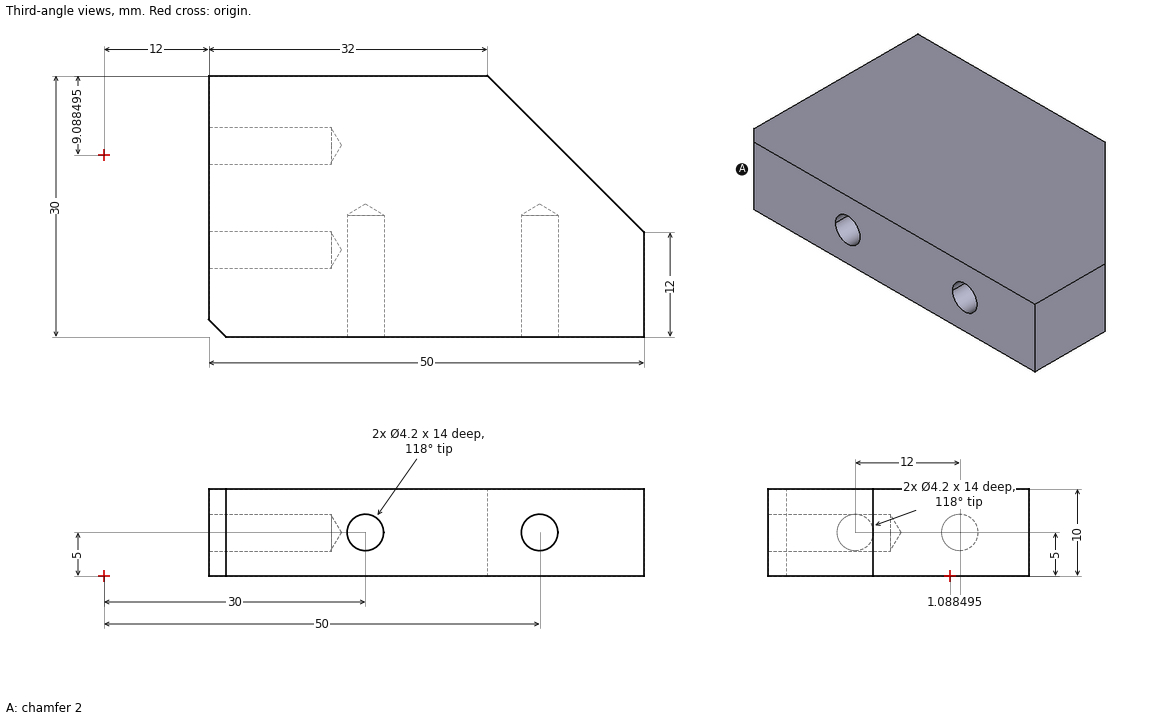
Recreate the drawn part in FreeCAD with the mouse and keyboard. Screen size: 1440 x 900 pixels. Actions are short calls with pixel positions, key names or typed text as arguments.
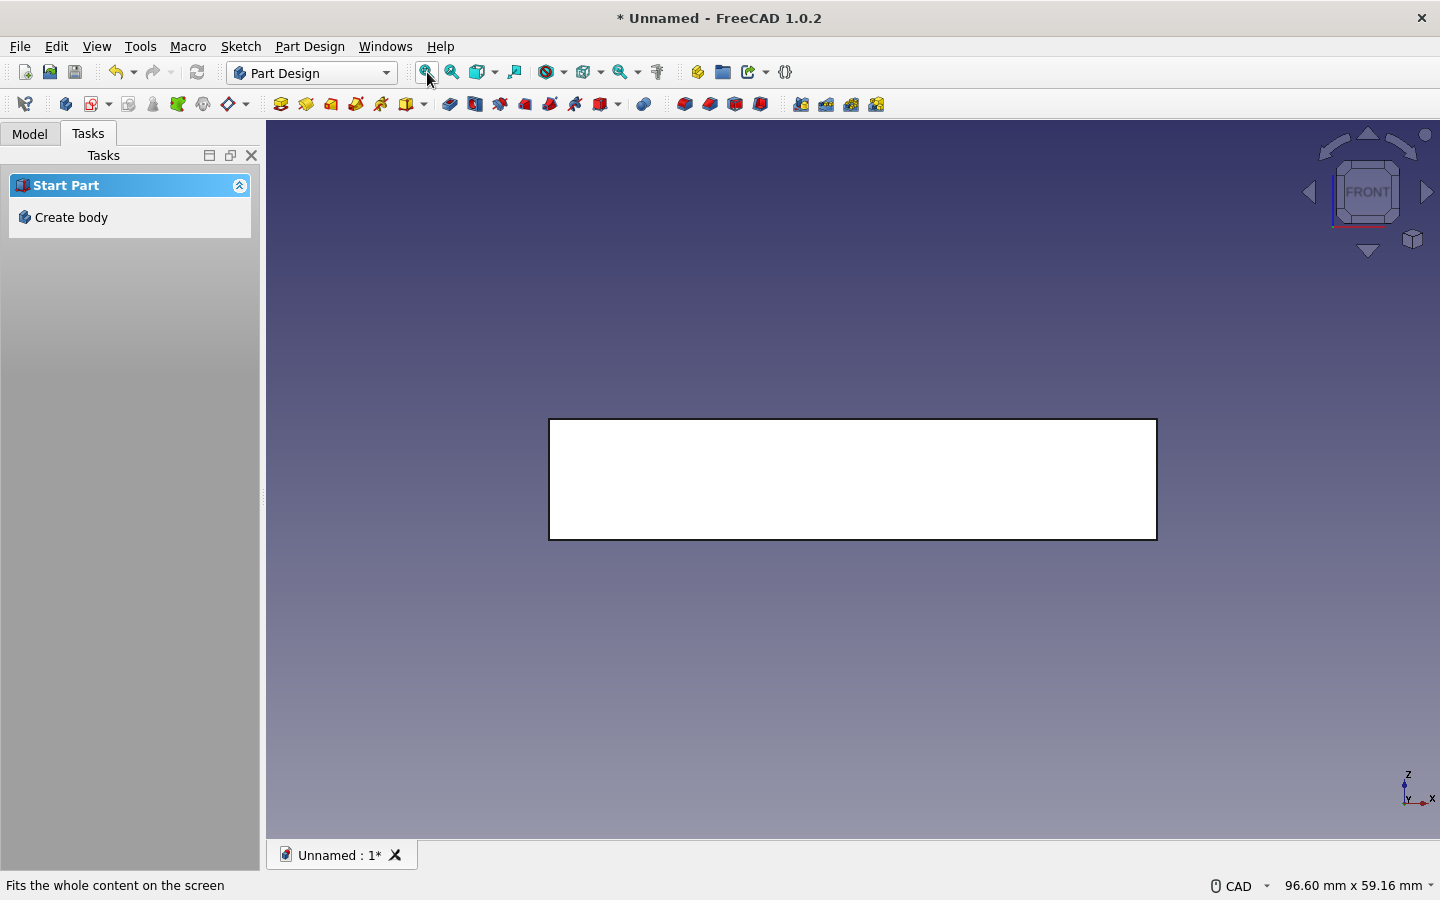
click(549, 479)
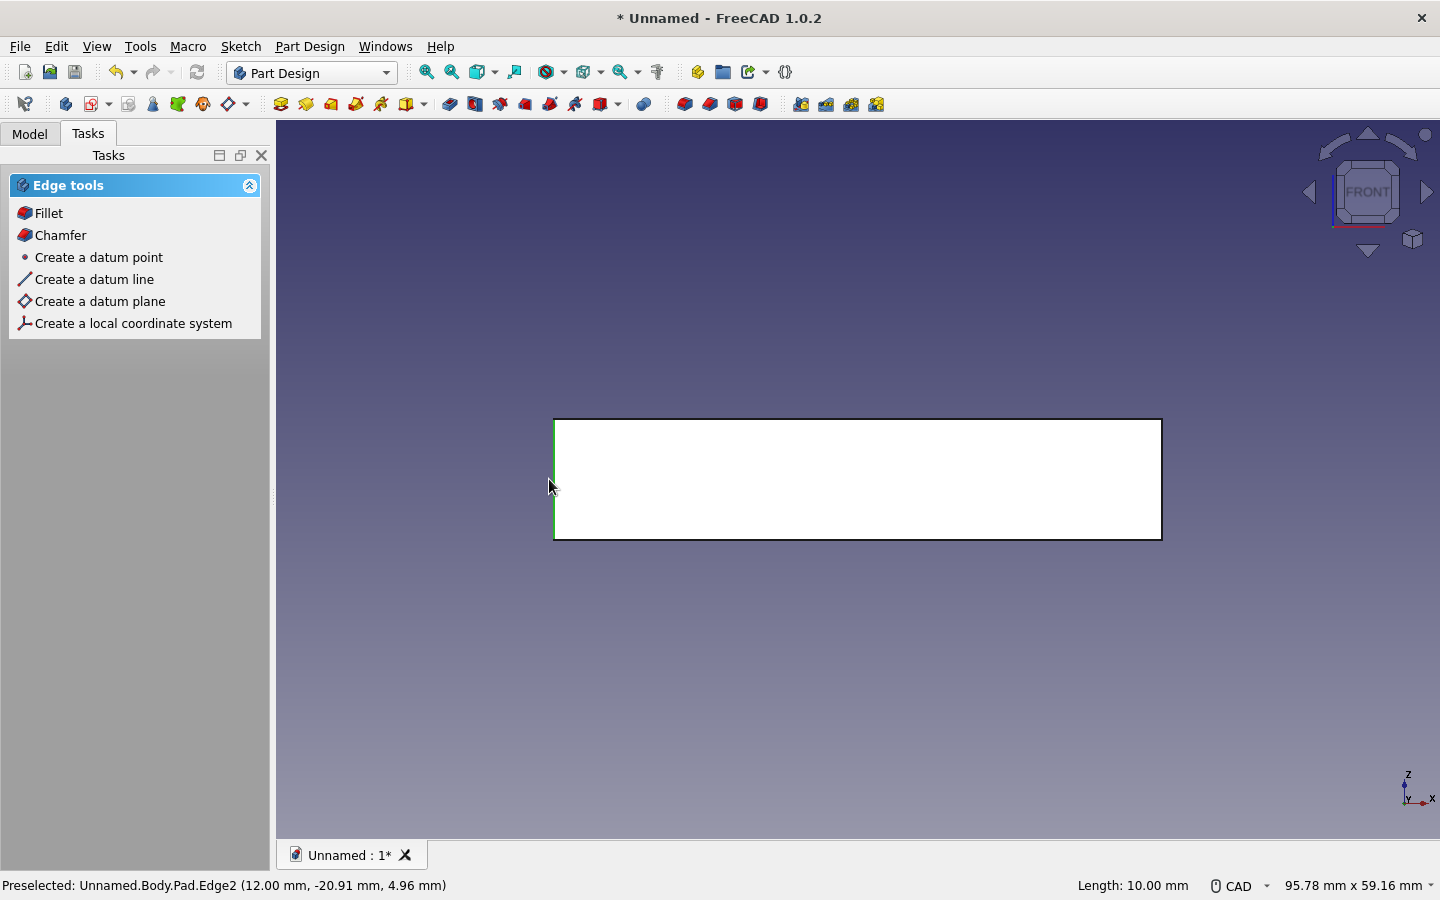
click(710, 104)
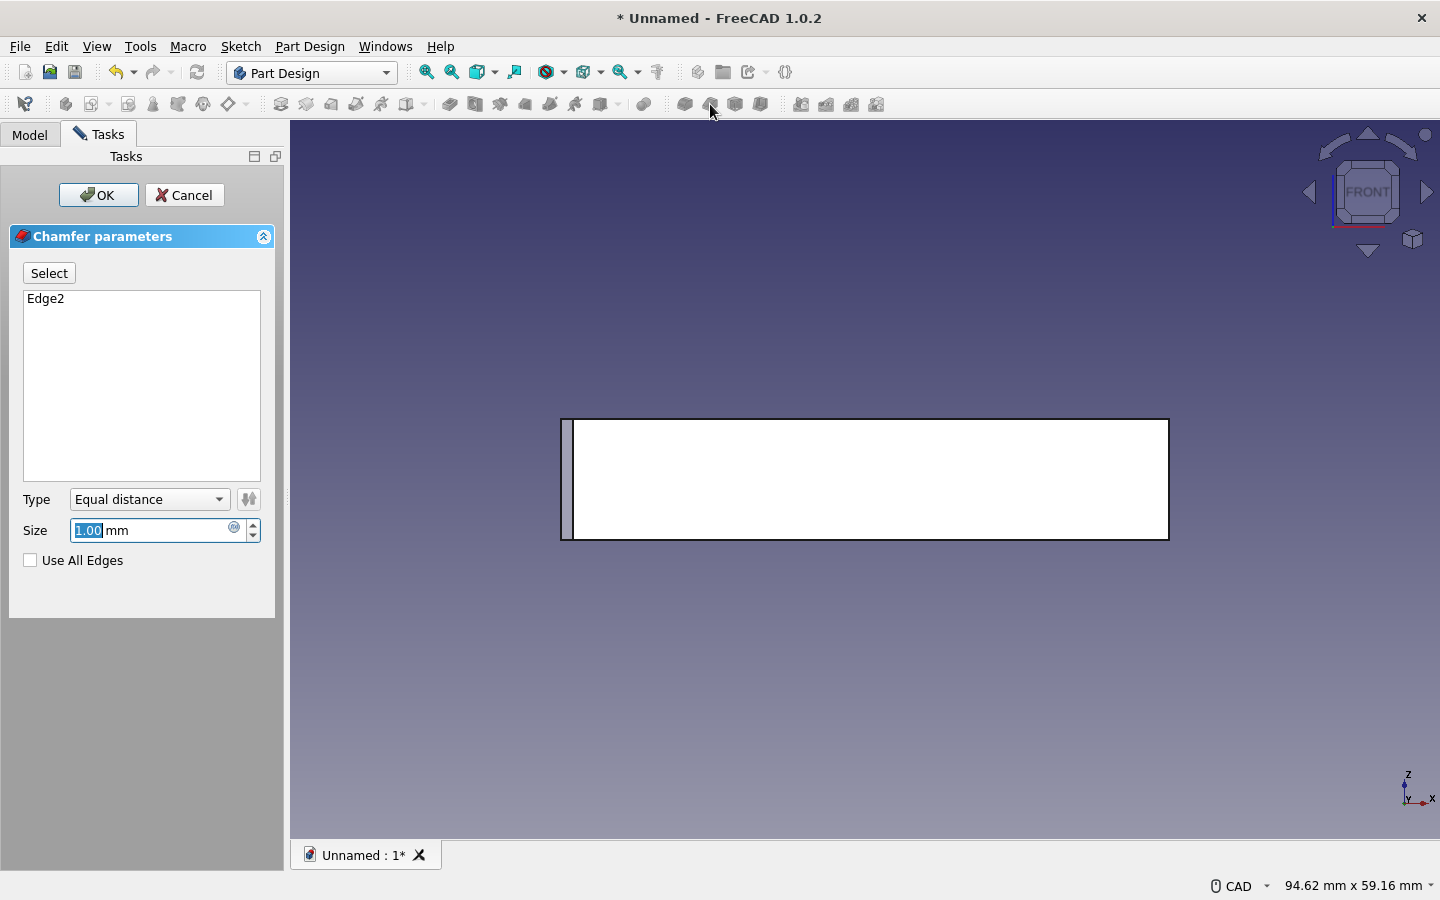
text(2)
key(Tab)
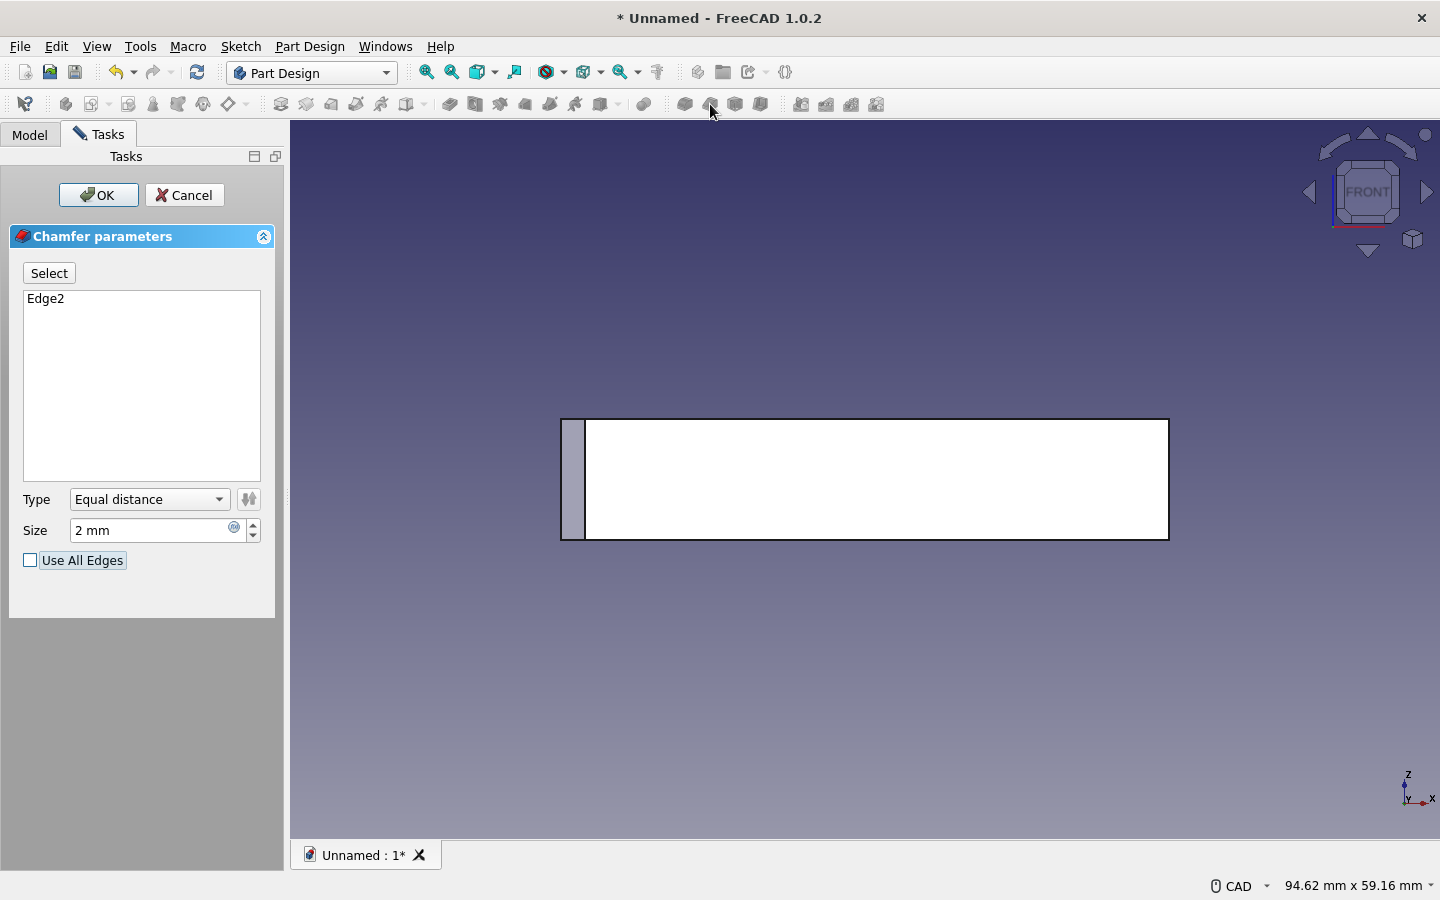
click(99, 195)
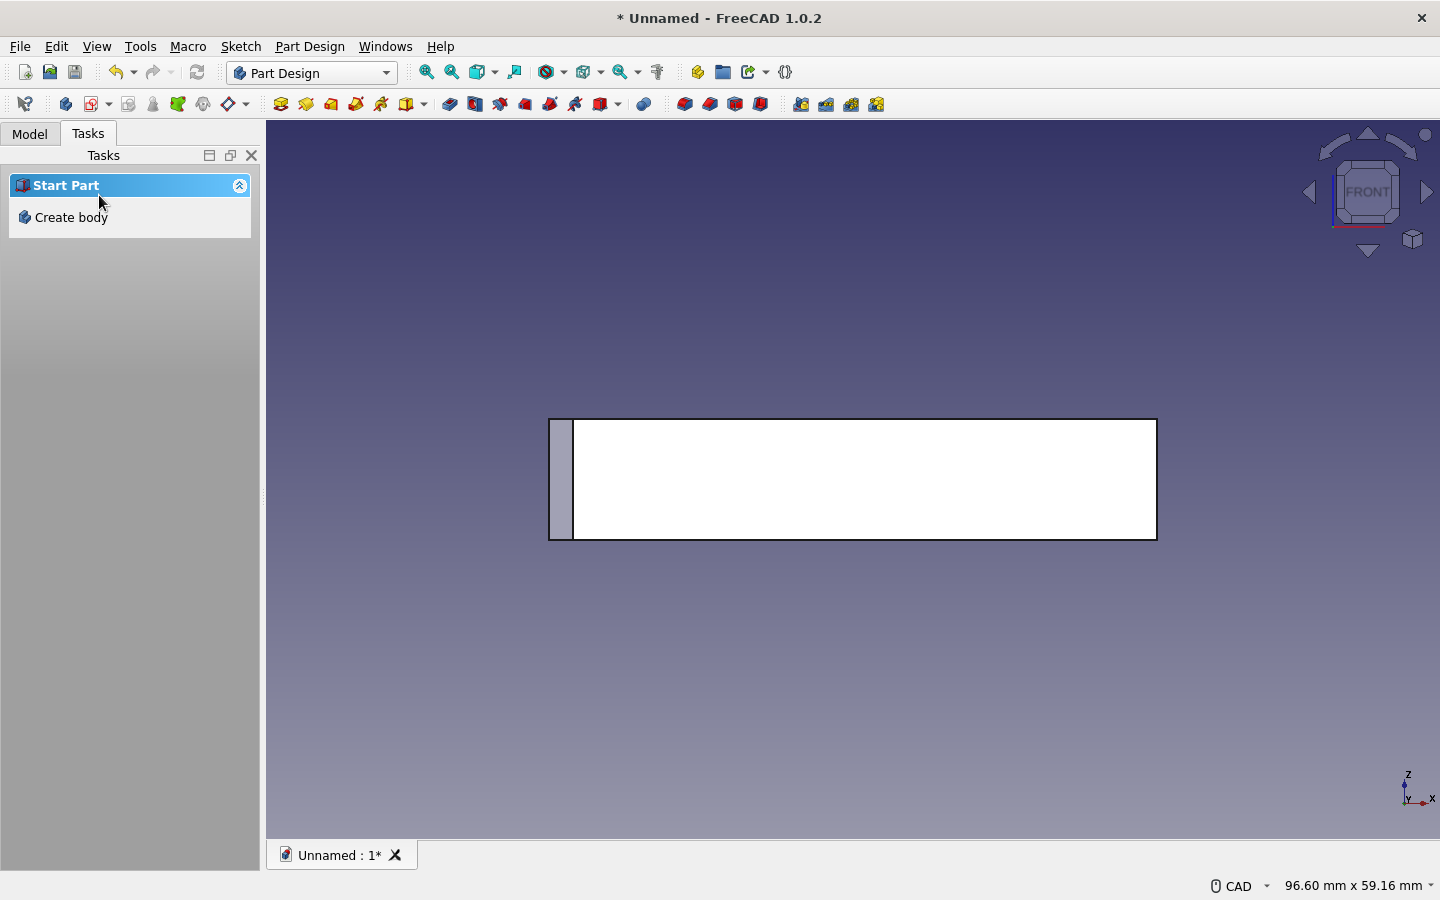
key(6)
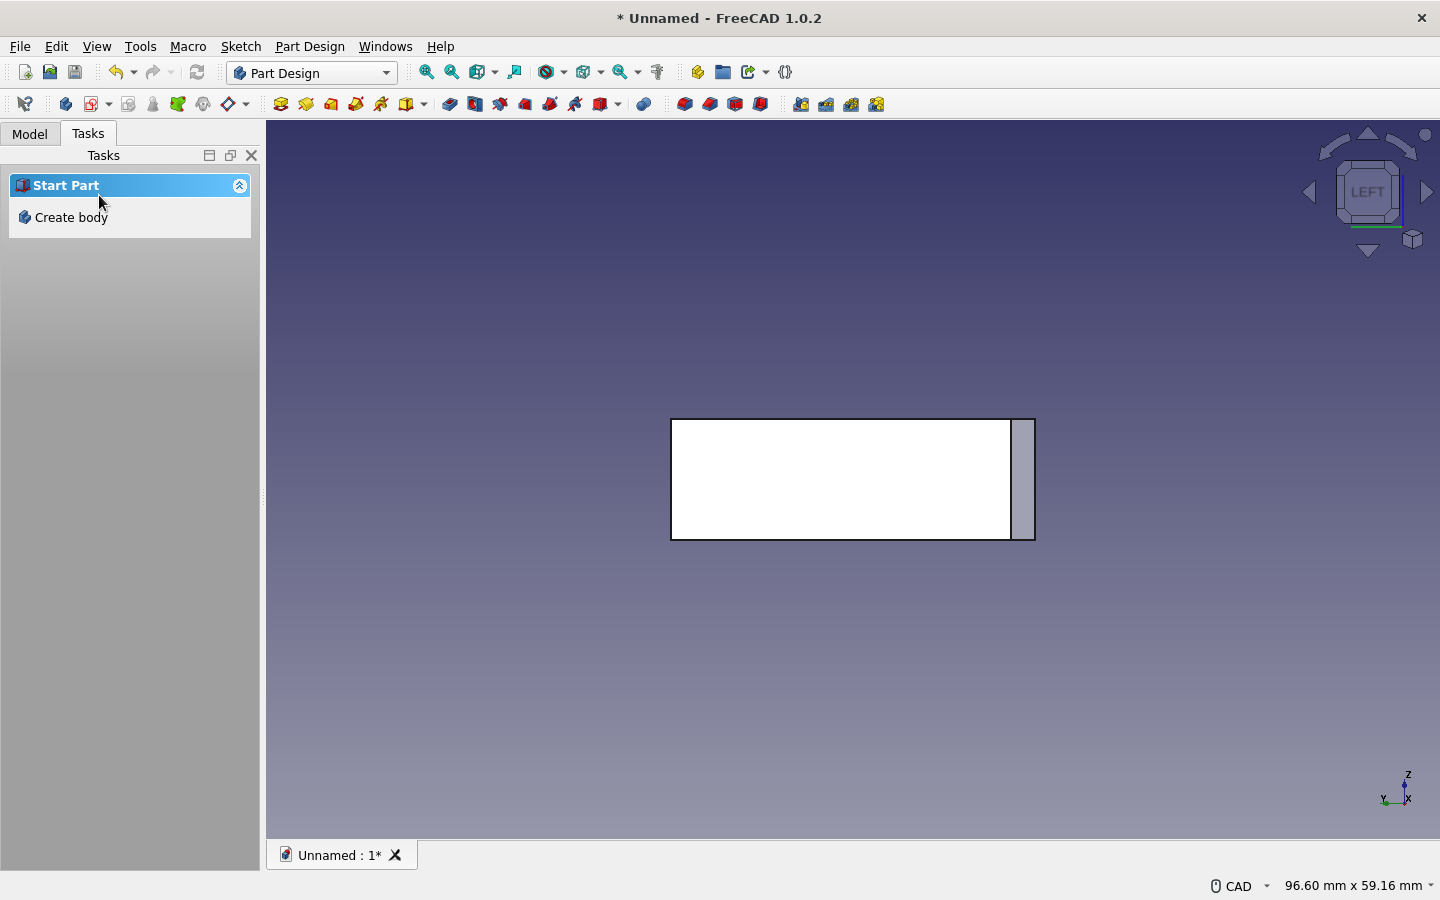
click(427, 72)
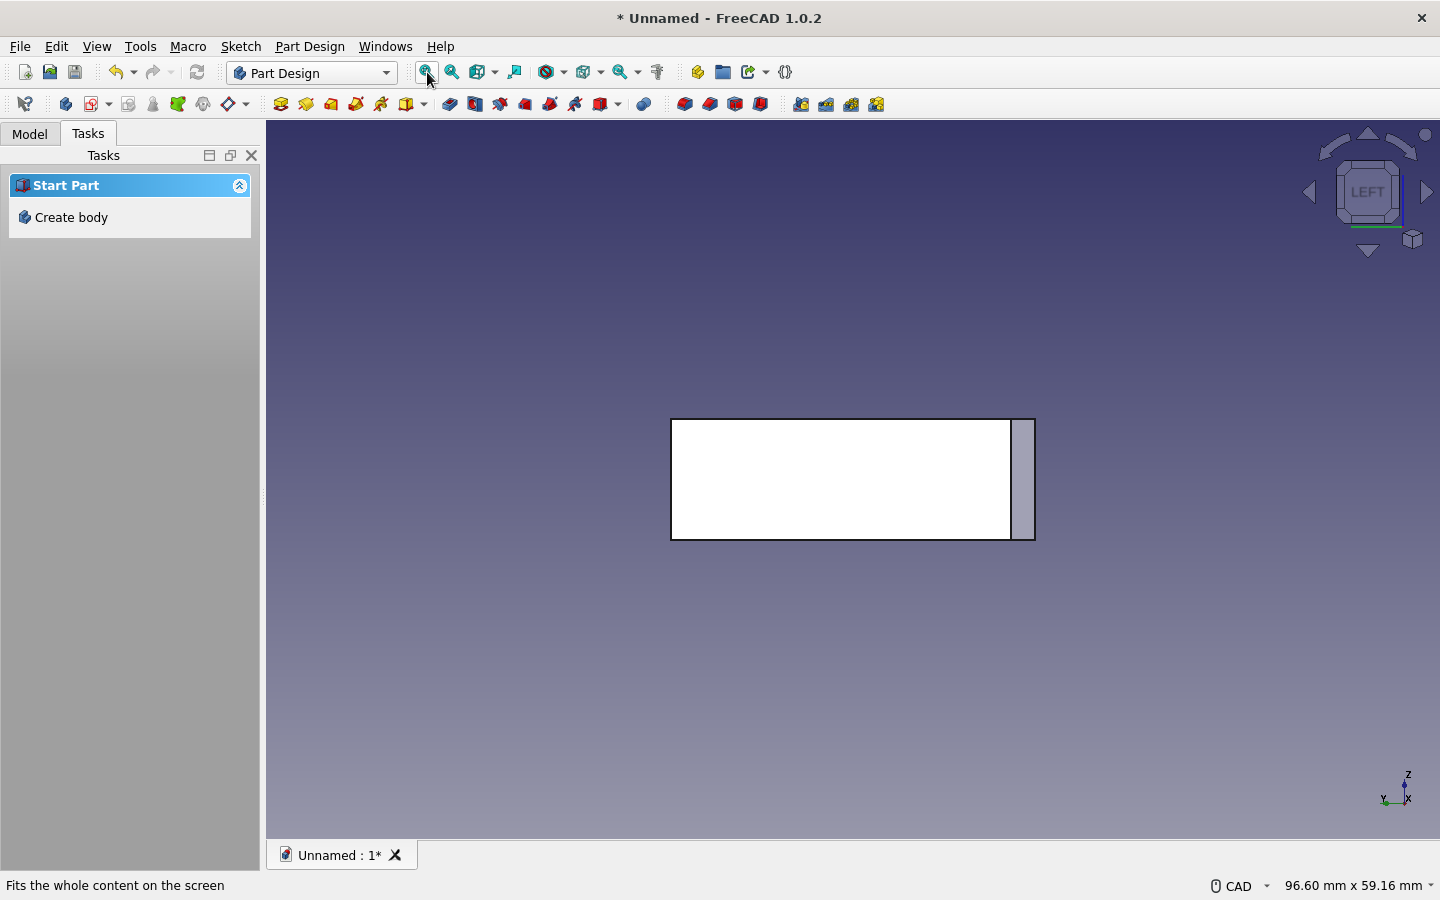
click(744, 478)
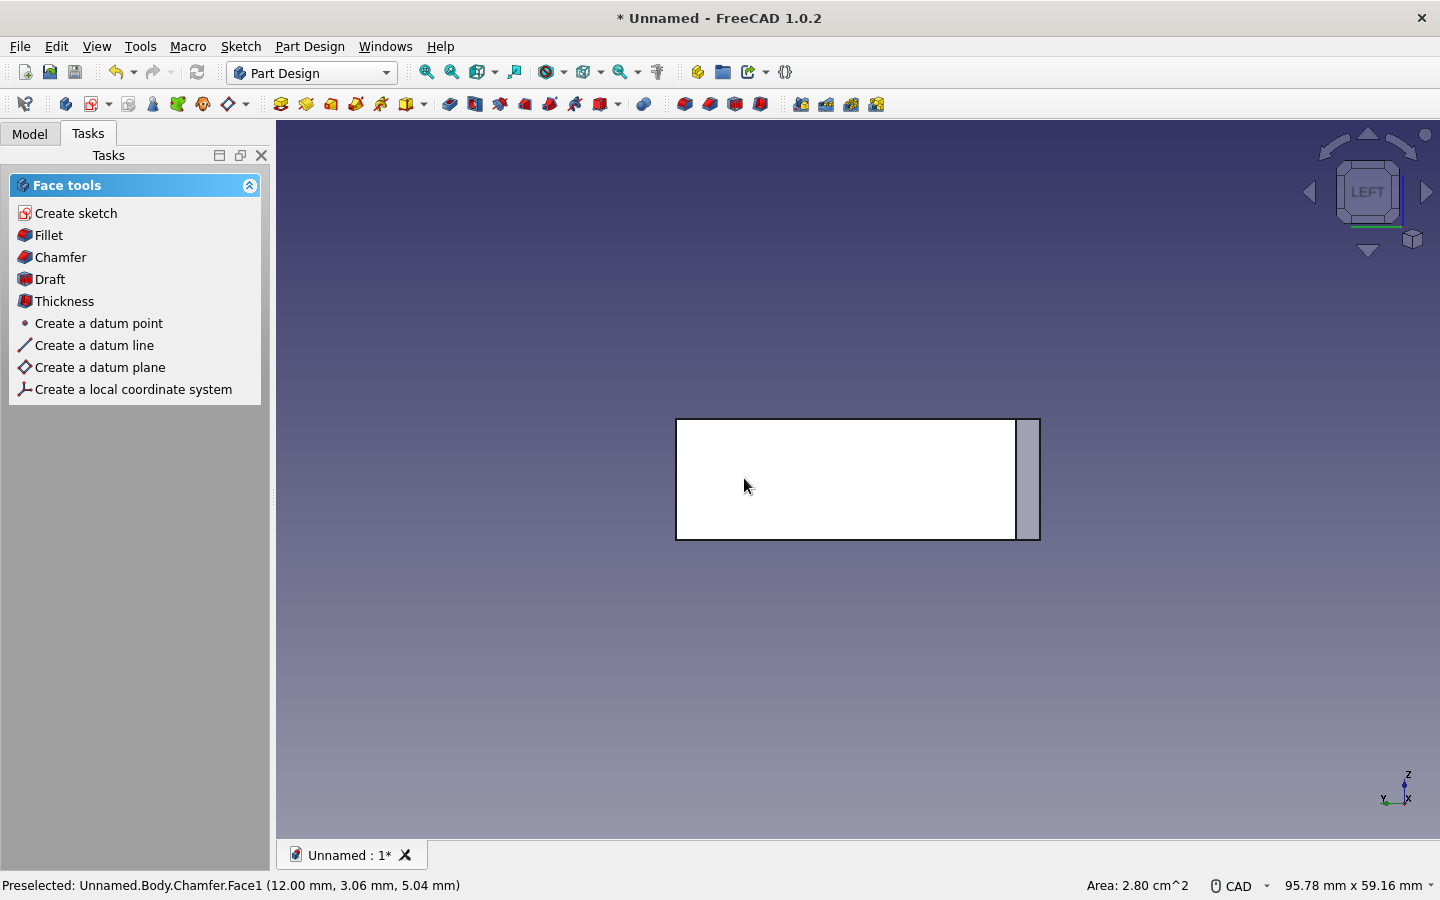
click(90, 104)